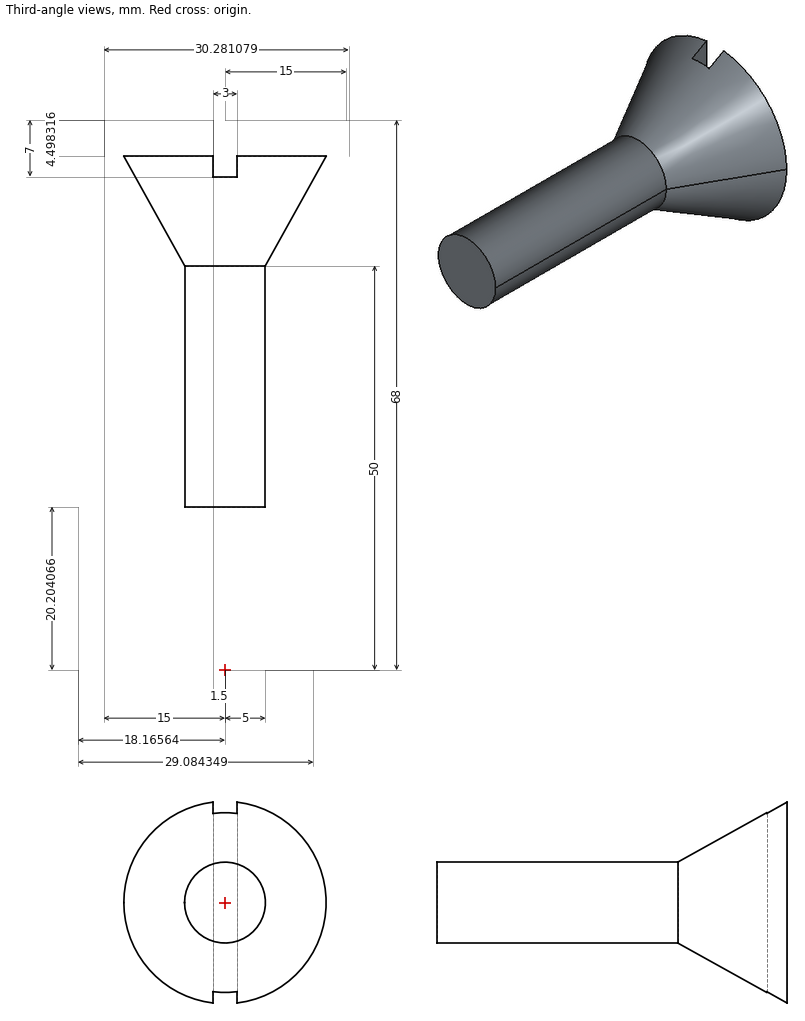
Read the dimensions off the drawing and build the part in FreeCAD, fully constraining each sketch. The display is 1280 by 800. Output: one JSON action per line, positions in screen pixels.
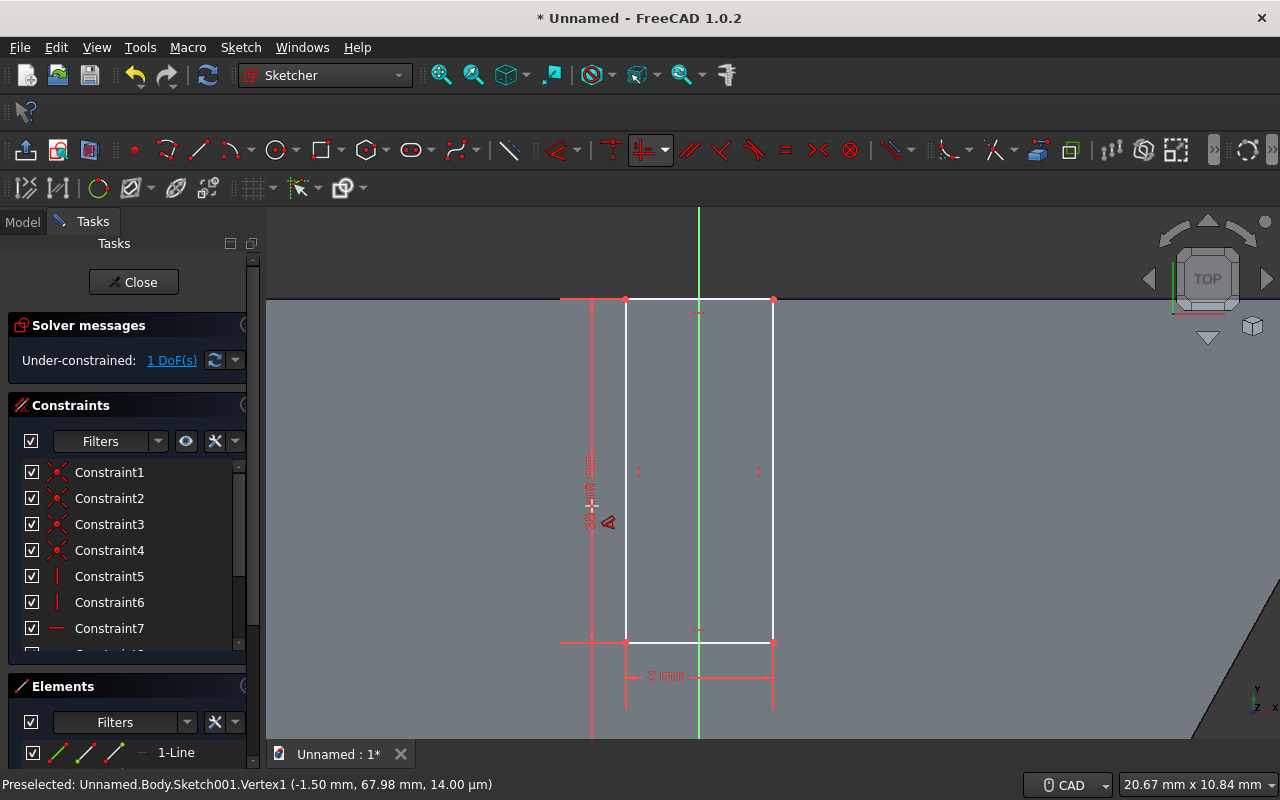
{"action": "left_click", "coordinate": [626, 299]}
{"action": "left_click", "coordinate": [663, 265]}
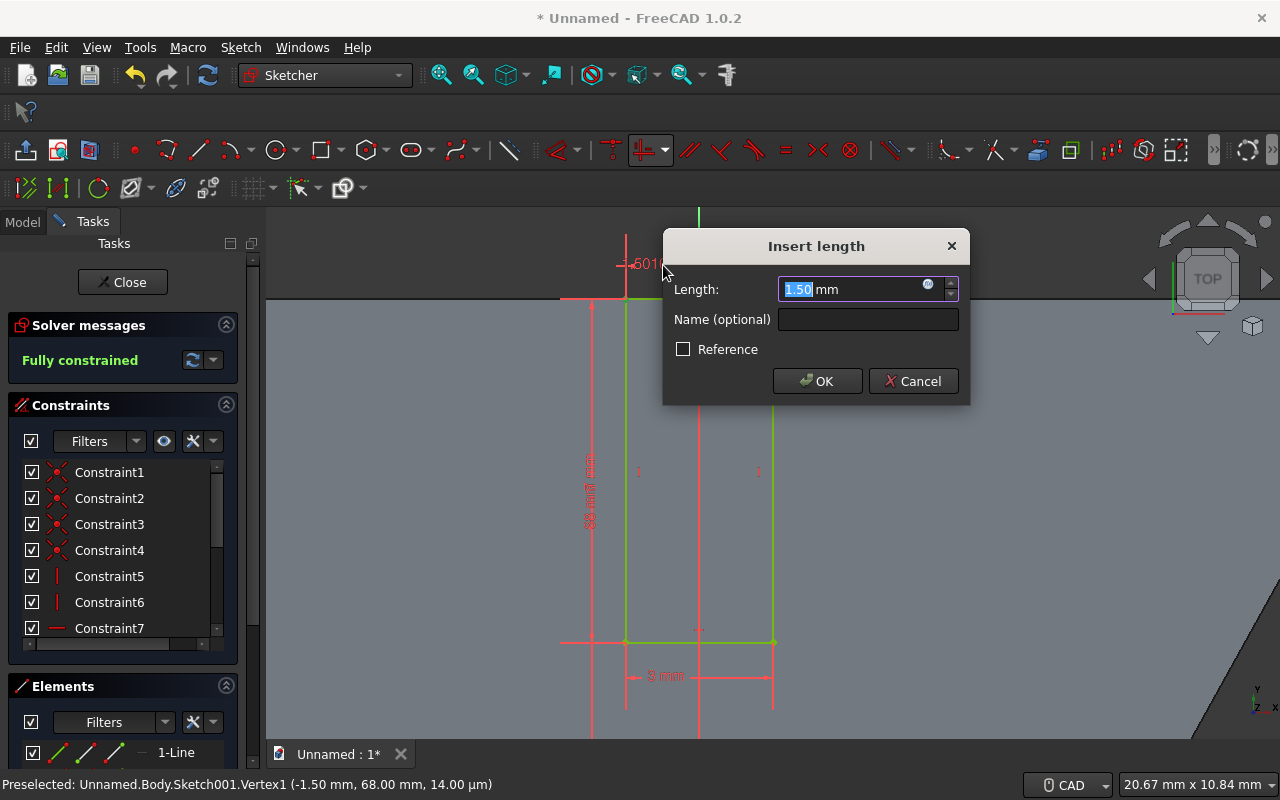
{"action": "type", "text": "1.5"}
{"action": "key", "text": "Return"}
{"action": "key", "text": "Escape"}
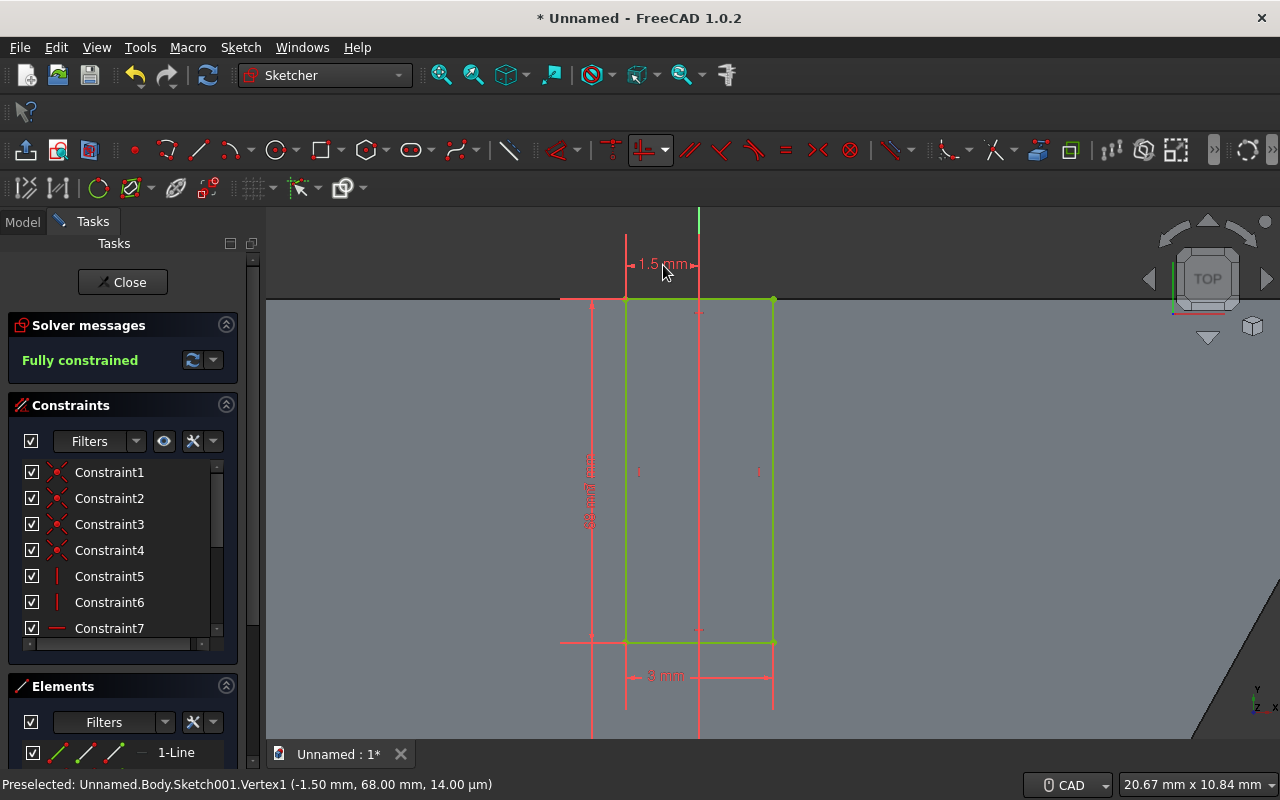
{"action": "left_click", "coordinate": [123, 282]}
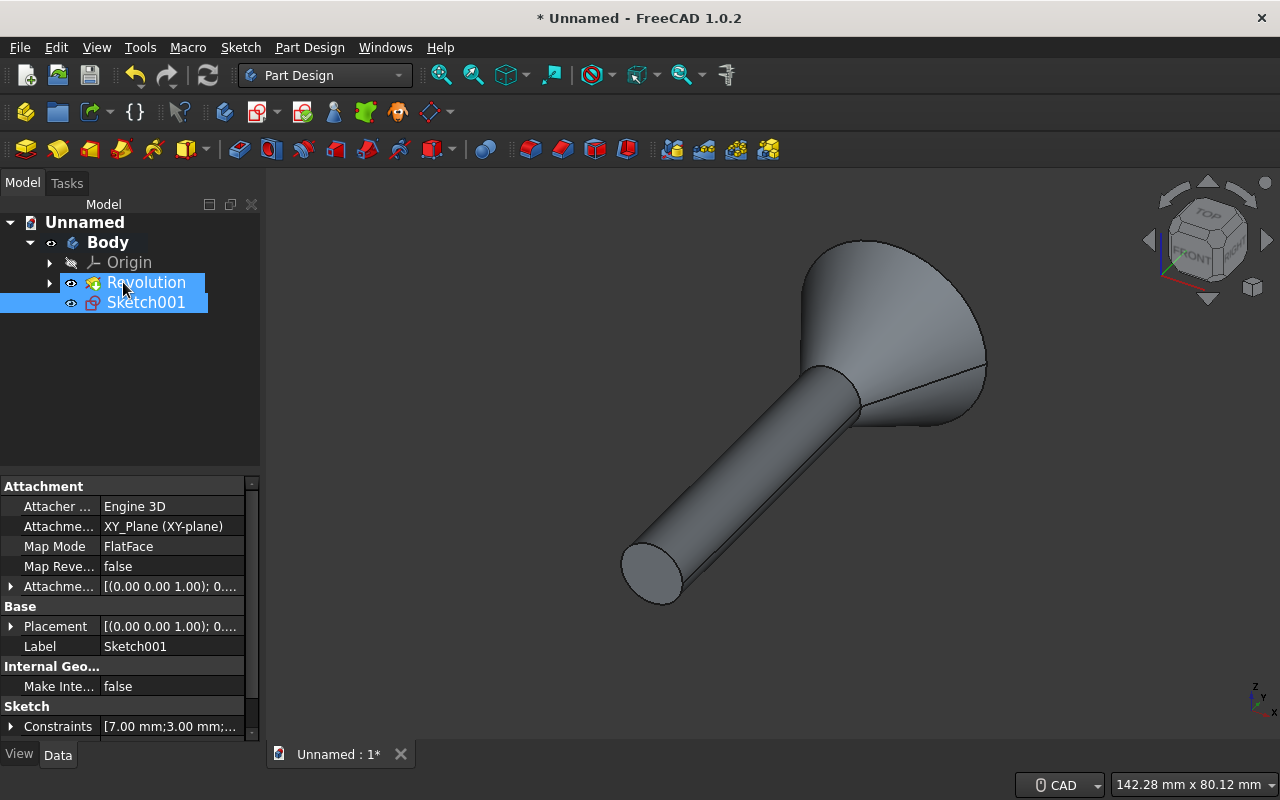
{"action": "left_click", "coordinate": [240, 150]}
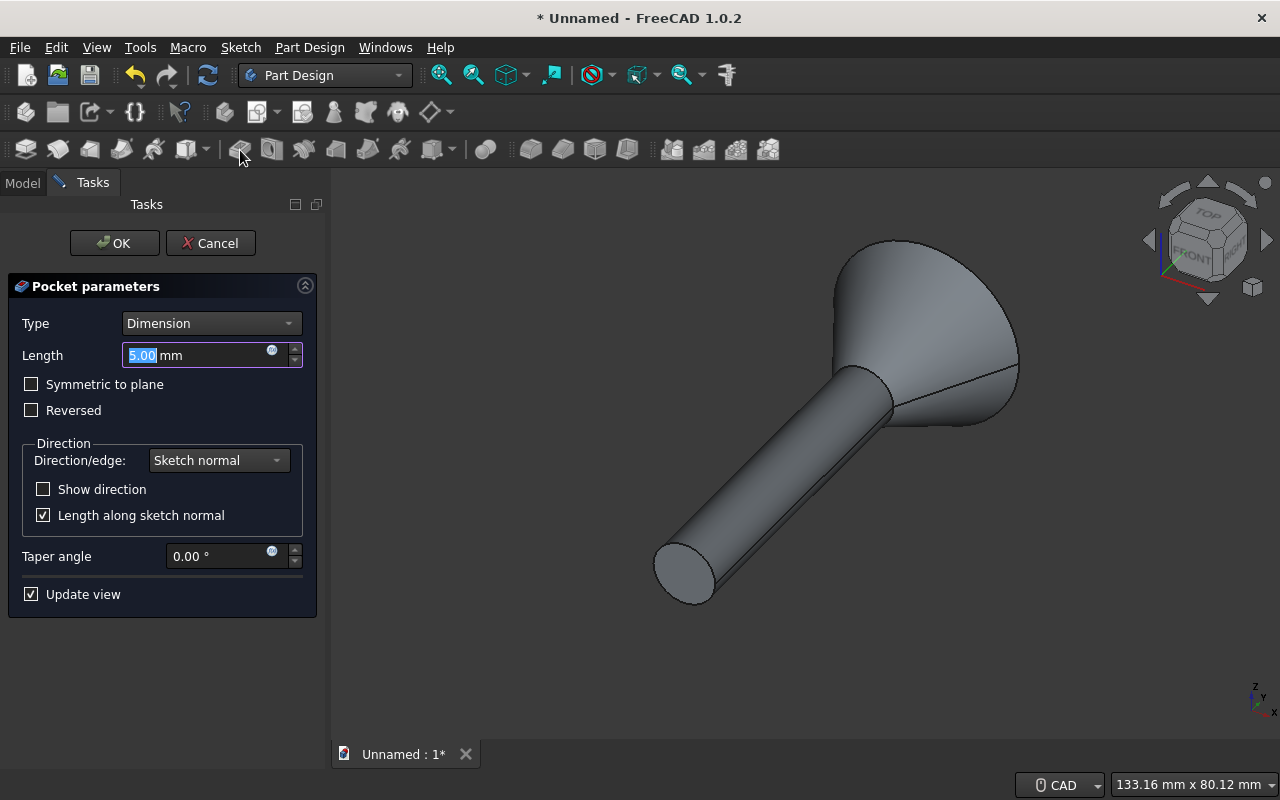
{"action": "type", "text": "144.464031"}
{"action": "key", "text": "Tab"}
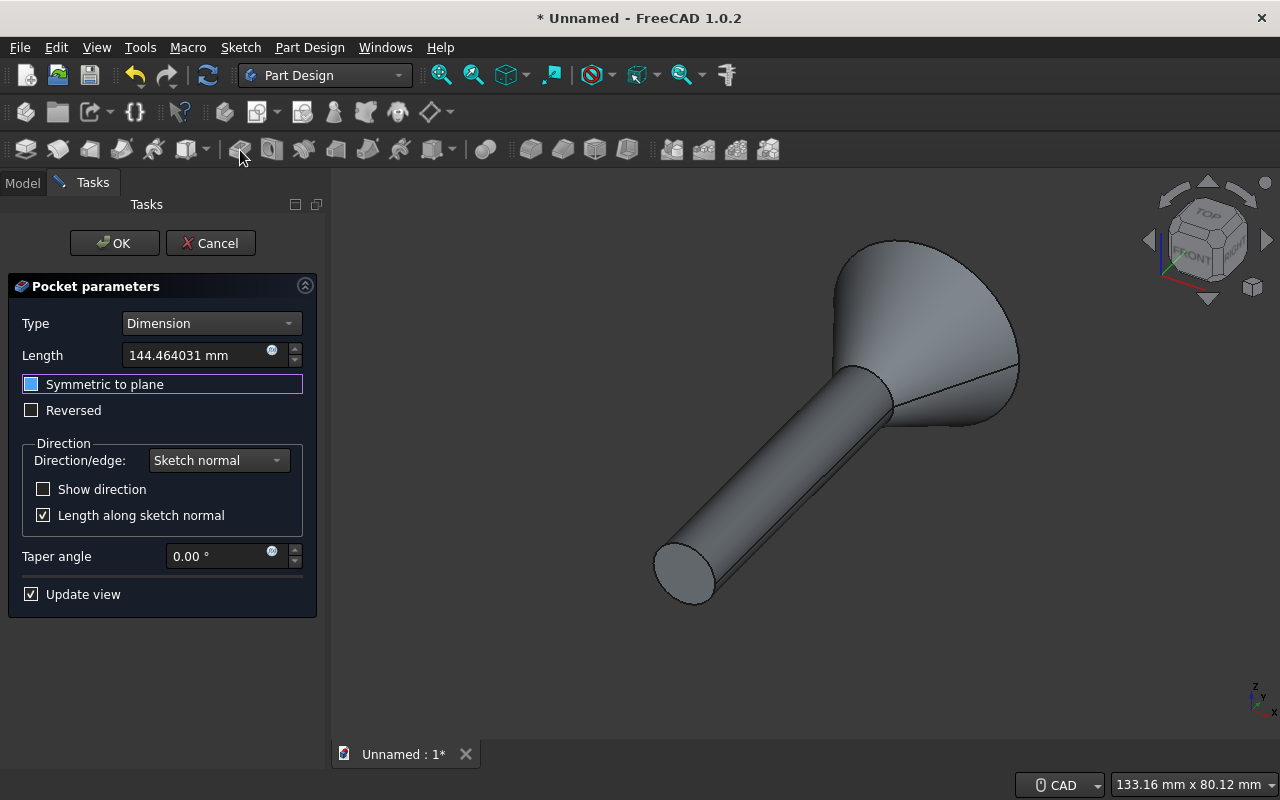
{"action": "left_click", "coordinate": [30, 384]}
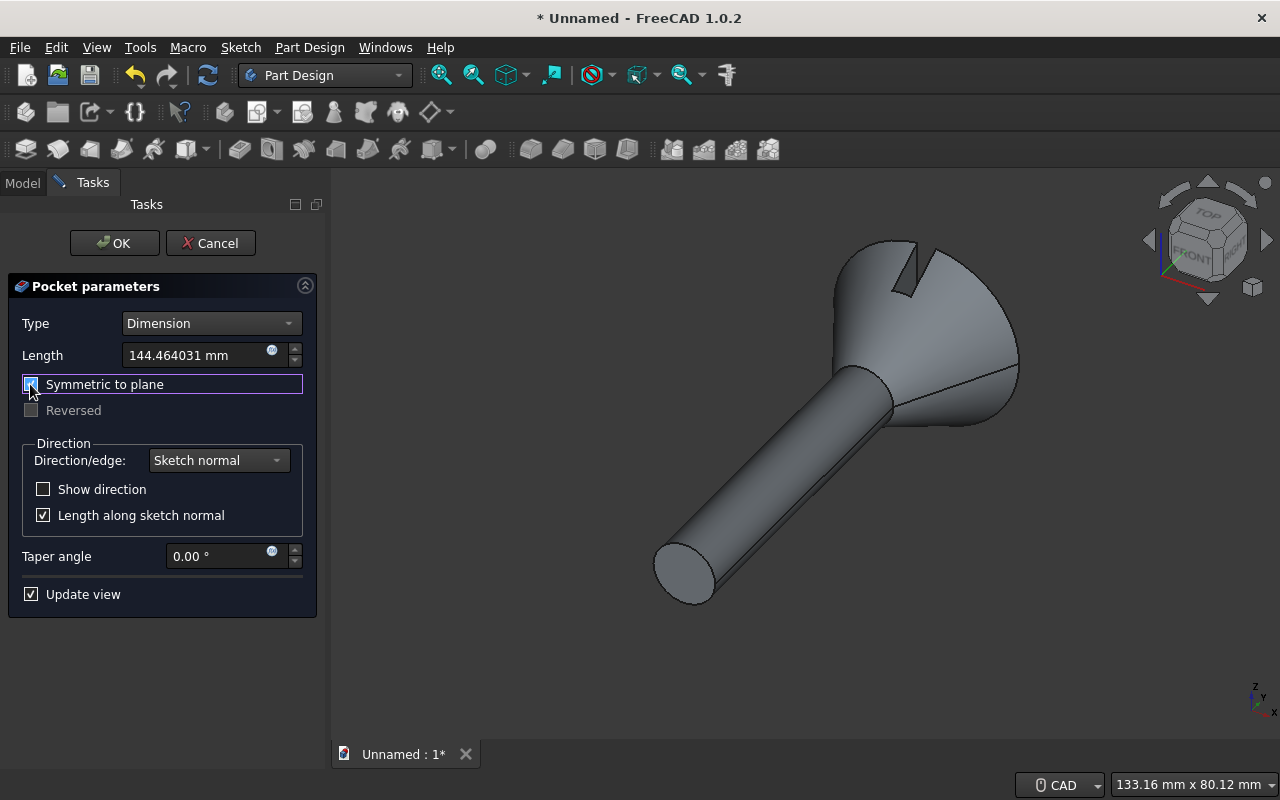
{"action": "left_click", "coordinate": [115, 243]}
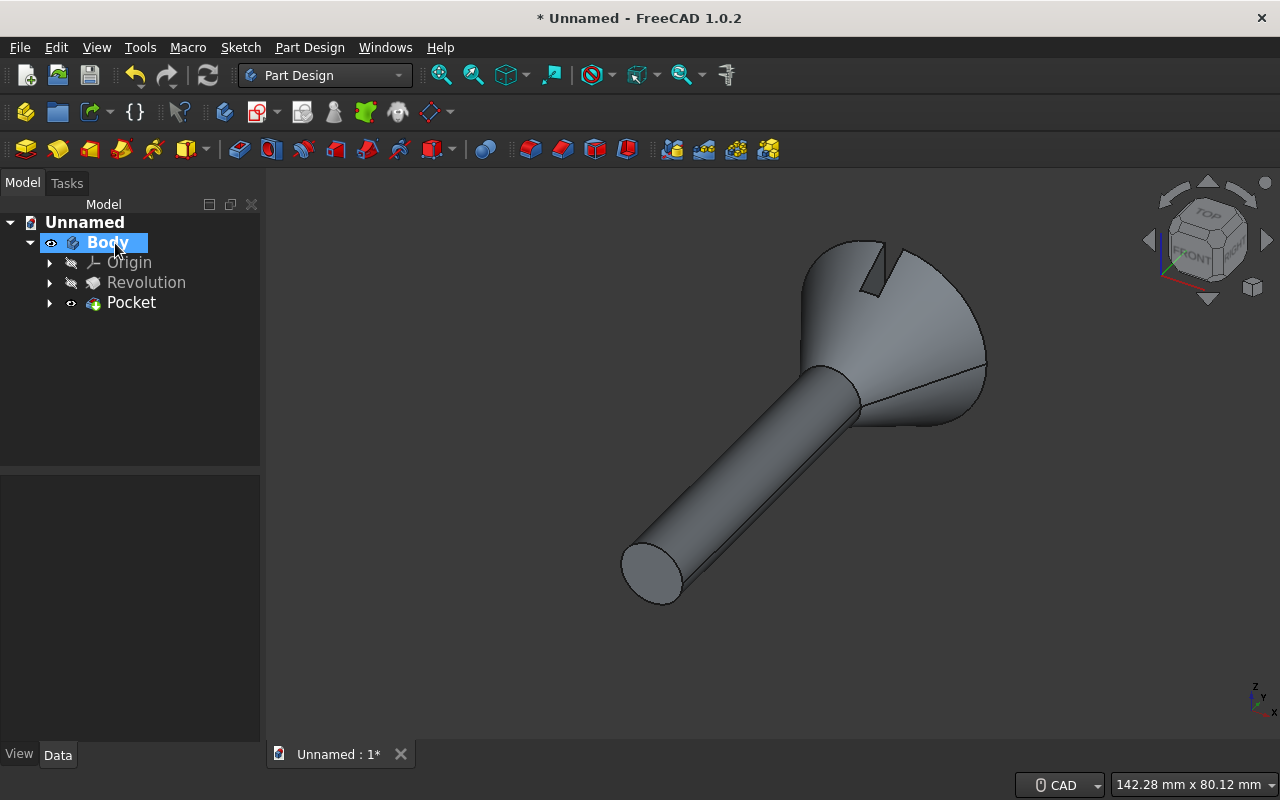
{"action": "left_click", "coordinate": [258, 112]}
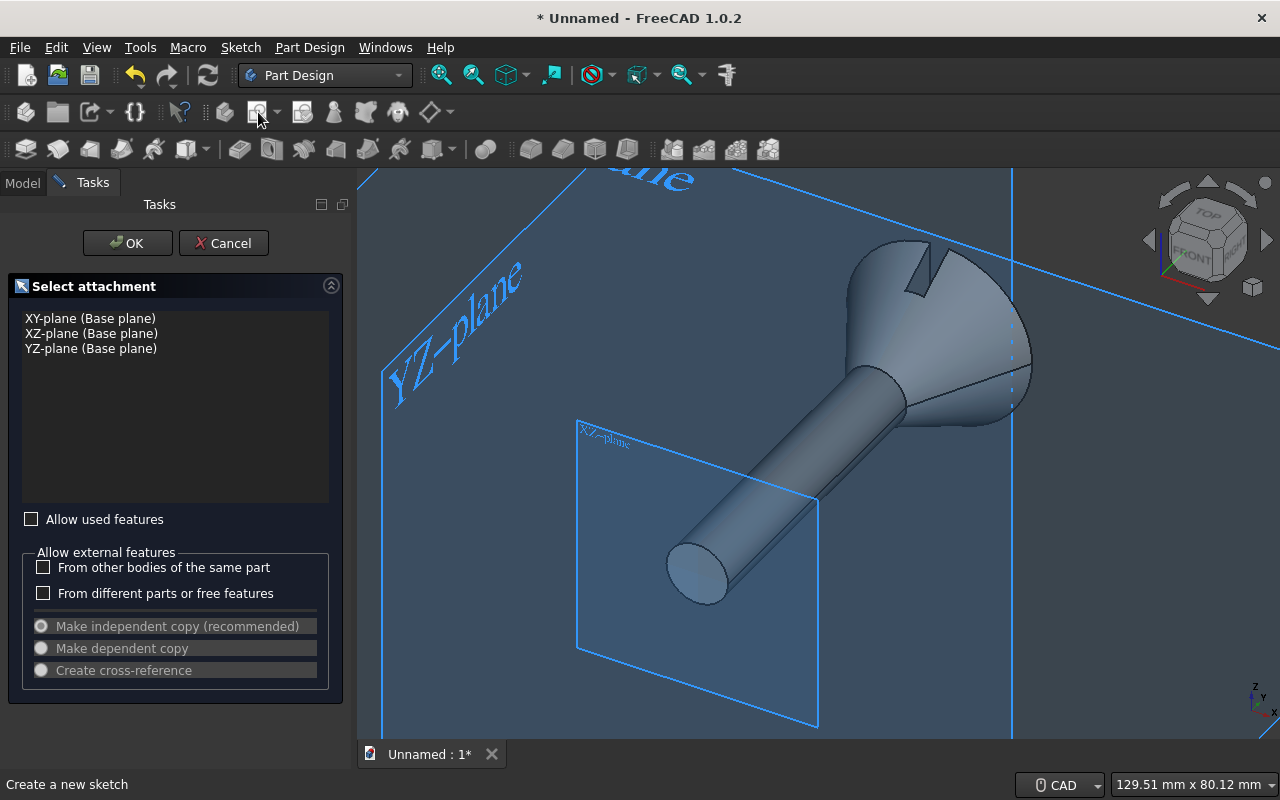
{"action": "left_click", "coordinate": [82, 318]}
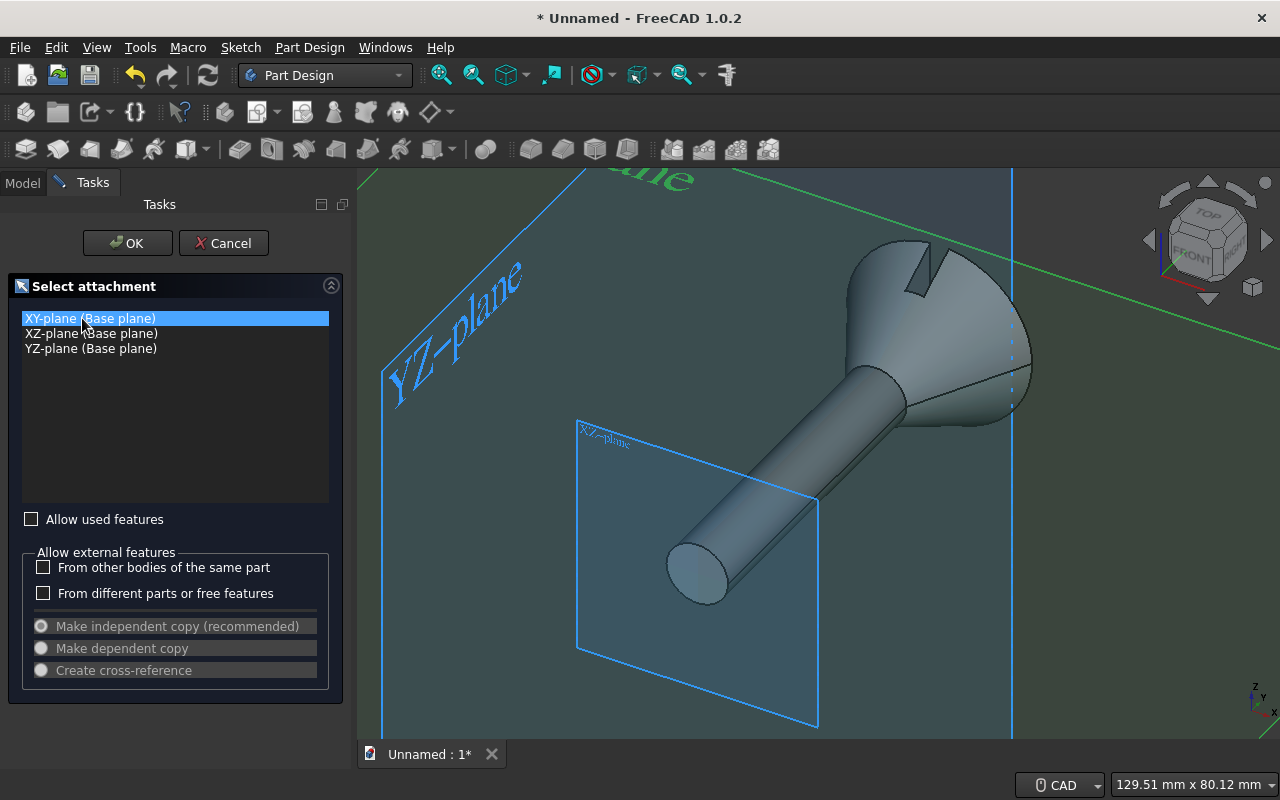
{"action": "left_click", "coordinate": [128, 243]}